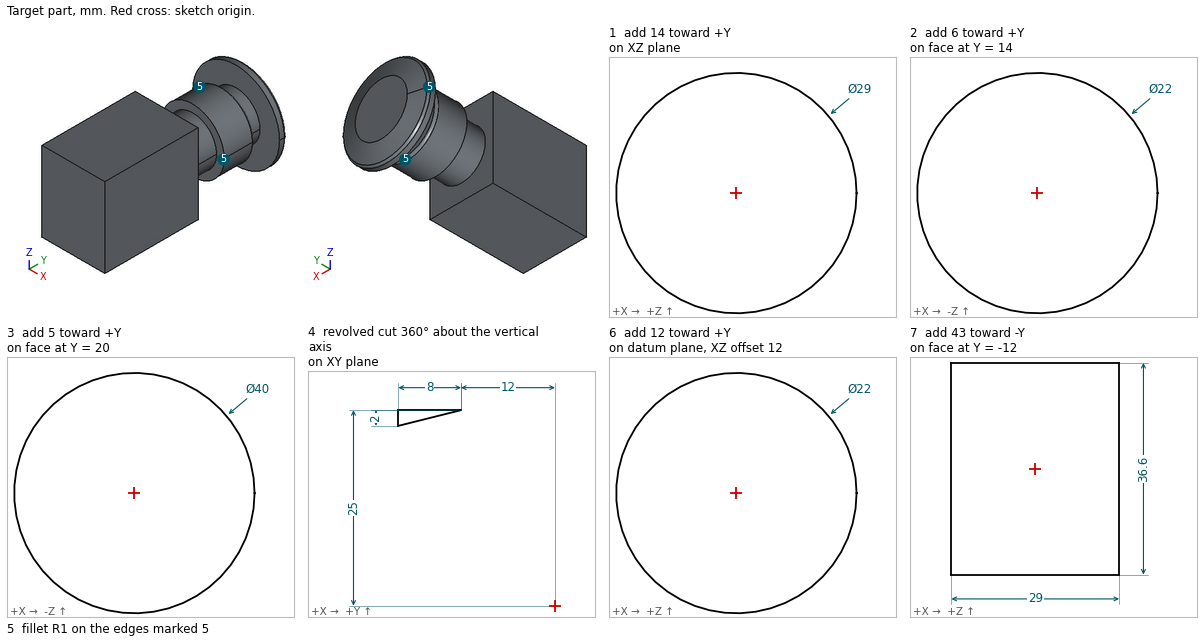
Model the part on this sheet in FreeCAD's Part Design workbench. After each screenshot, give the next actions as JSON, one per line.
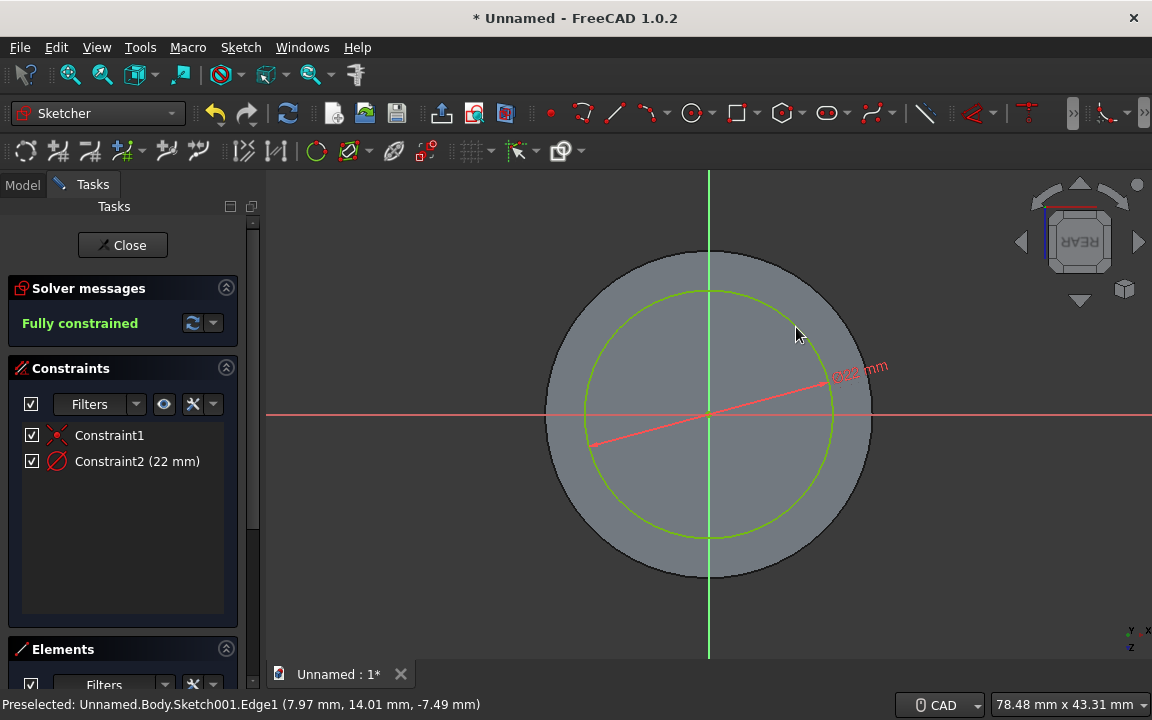
{"action": "left_click", "coordinate": [123, 245]}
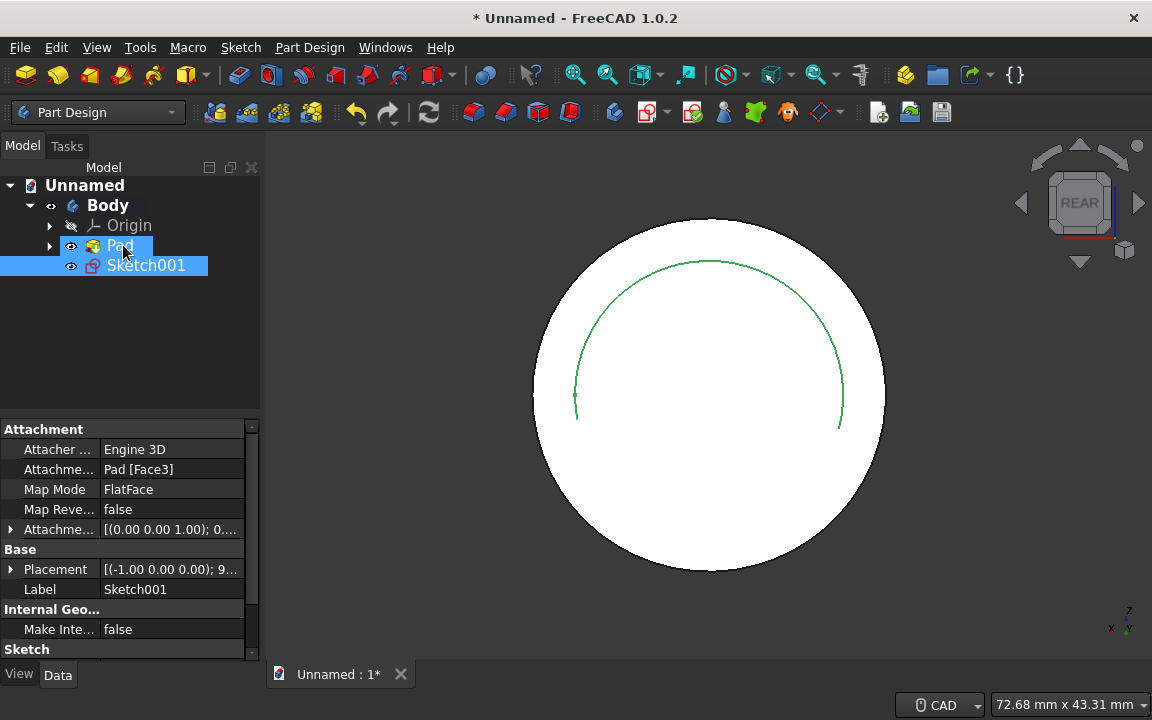
{"action": "left_click", "coordinate": [26, 76]}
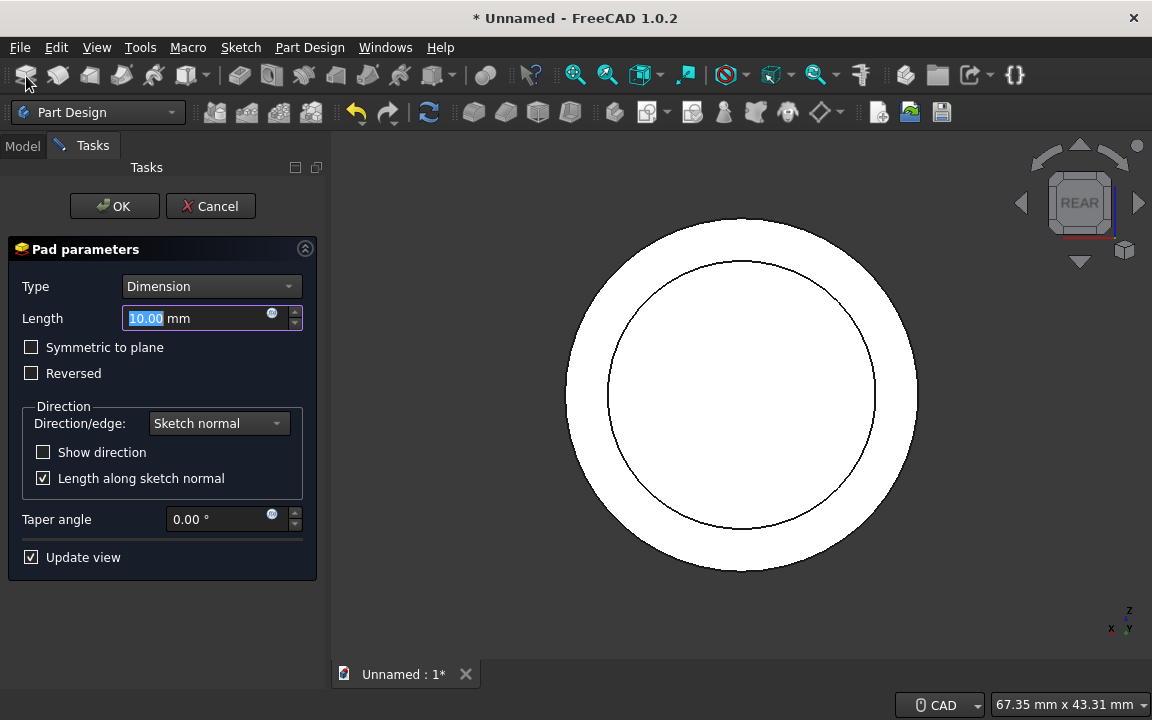
{"action": "type", "text": "6"}
{"action": "key", "text": "Tab"}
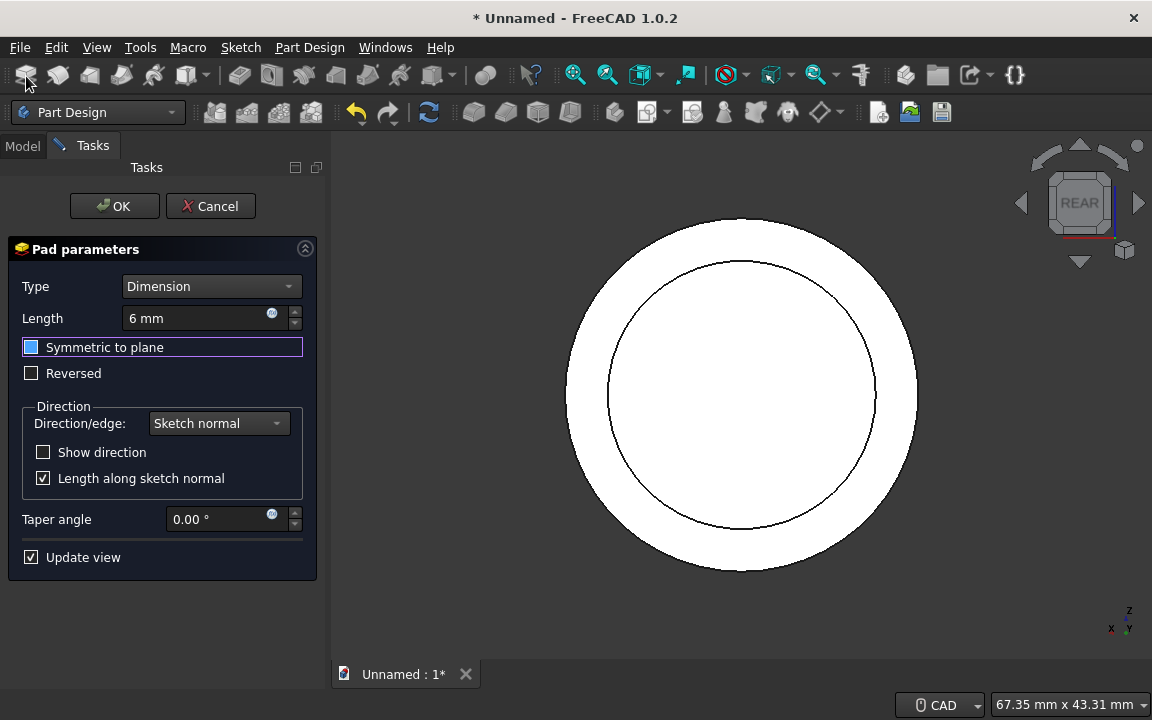
{"action": "left_click", "coordinate": [115, 206]}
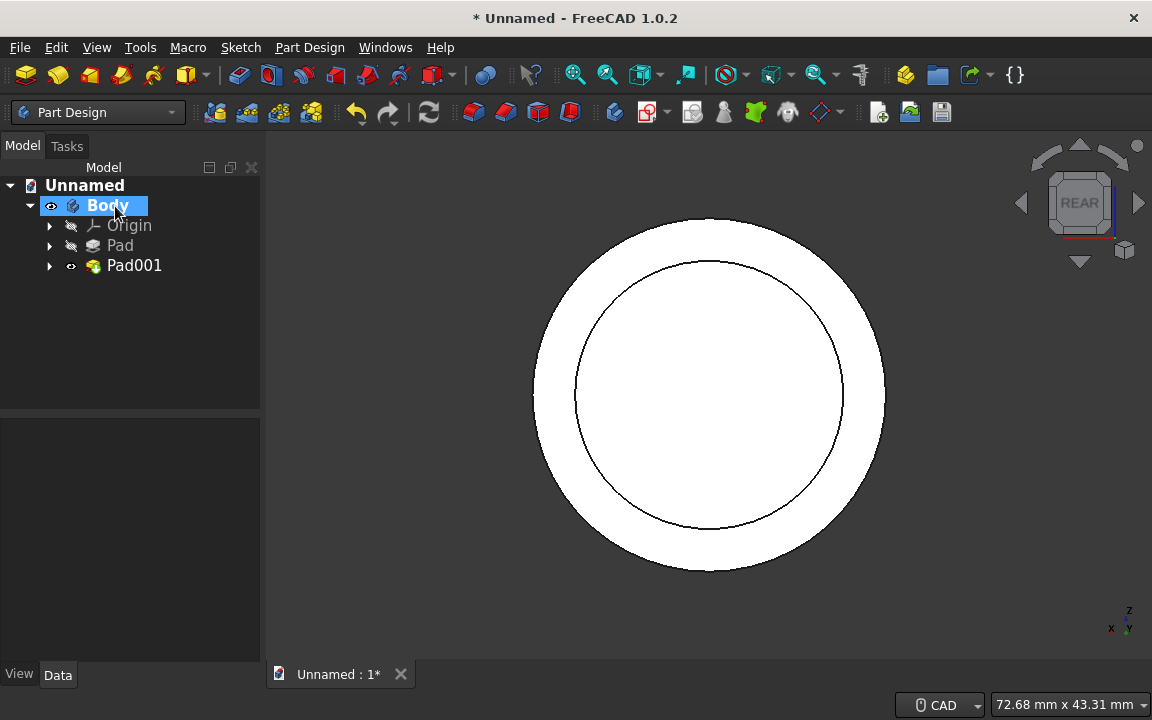
{"action": "left_click", "coordinate": [709, 394]}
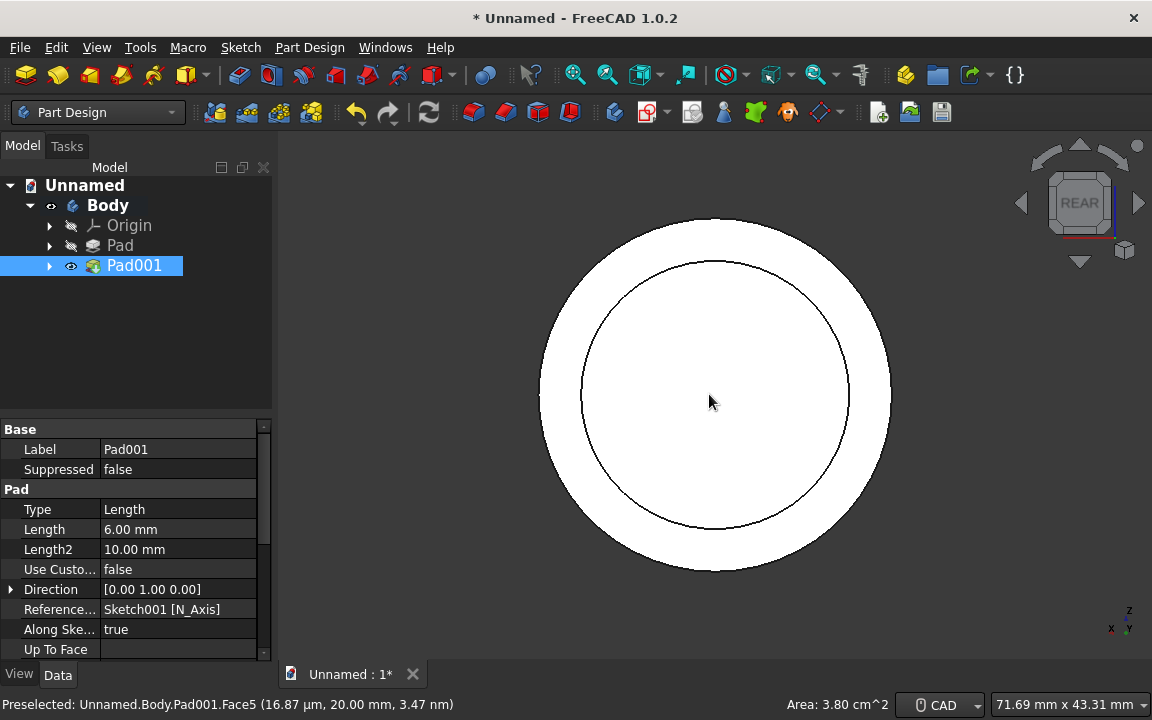
{"action": "left_click", "coordinate": [648, 112]}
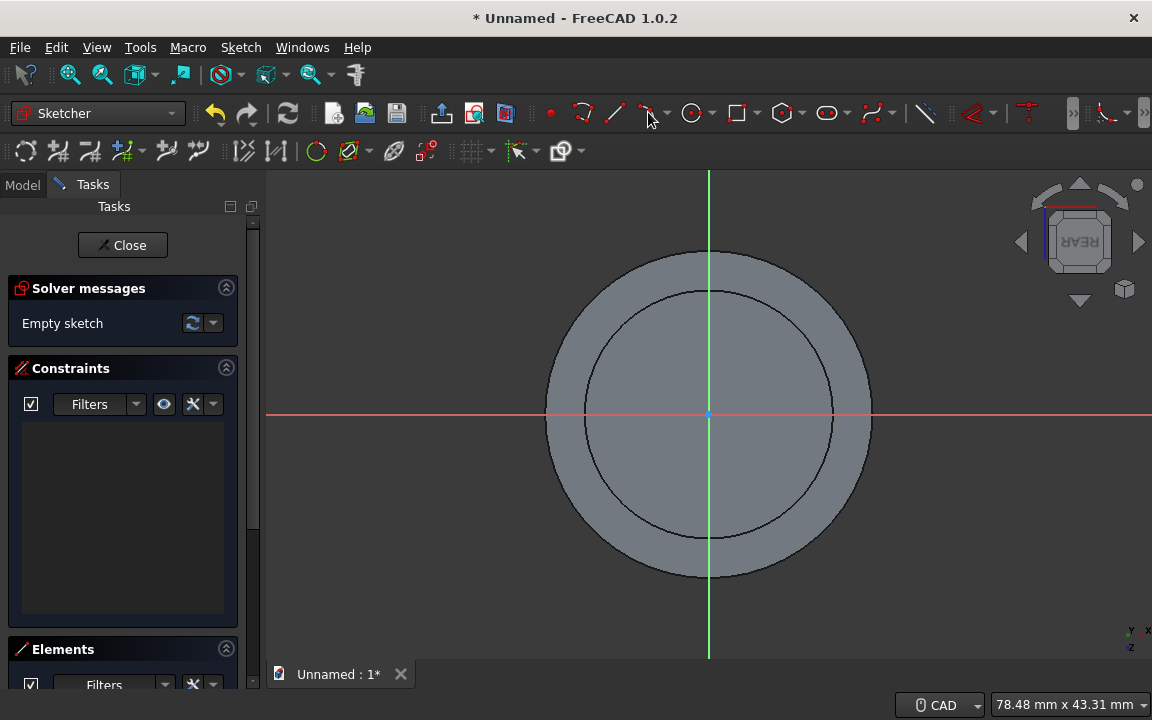
{"action": "scroll", "coordinate": [502, 415], "scroll_direction": "down", "scroll_amount": 2}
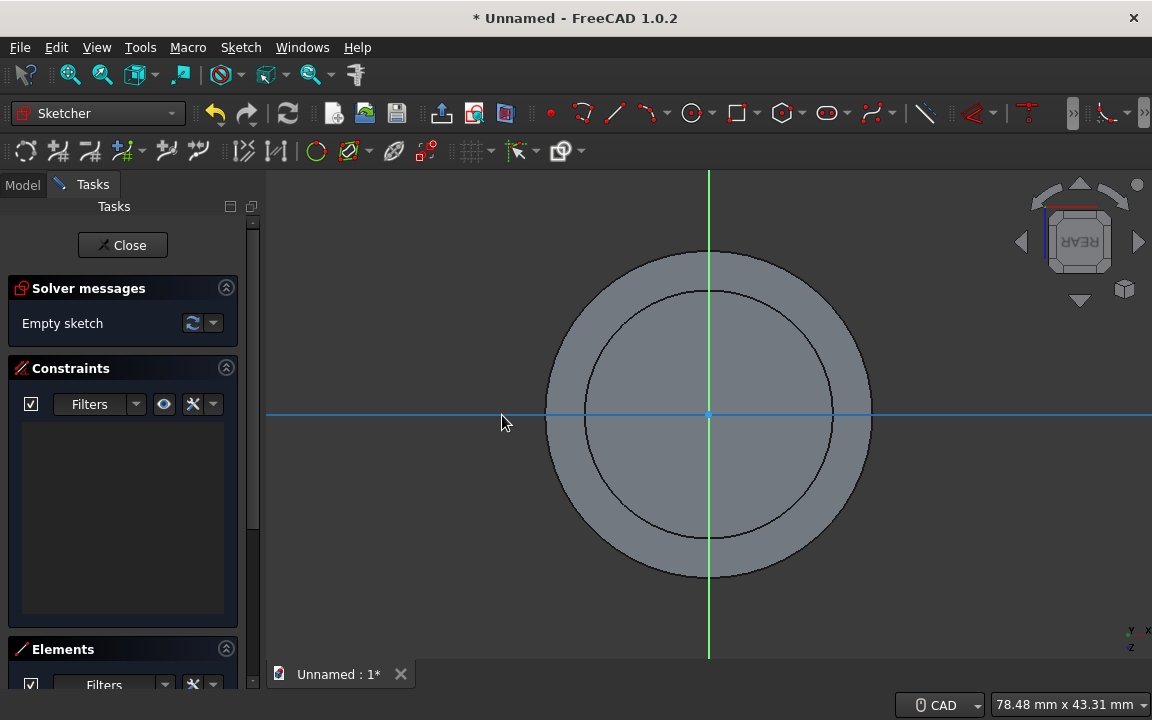
{"action": "key", "text": "g c"}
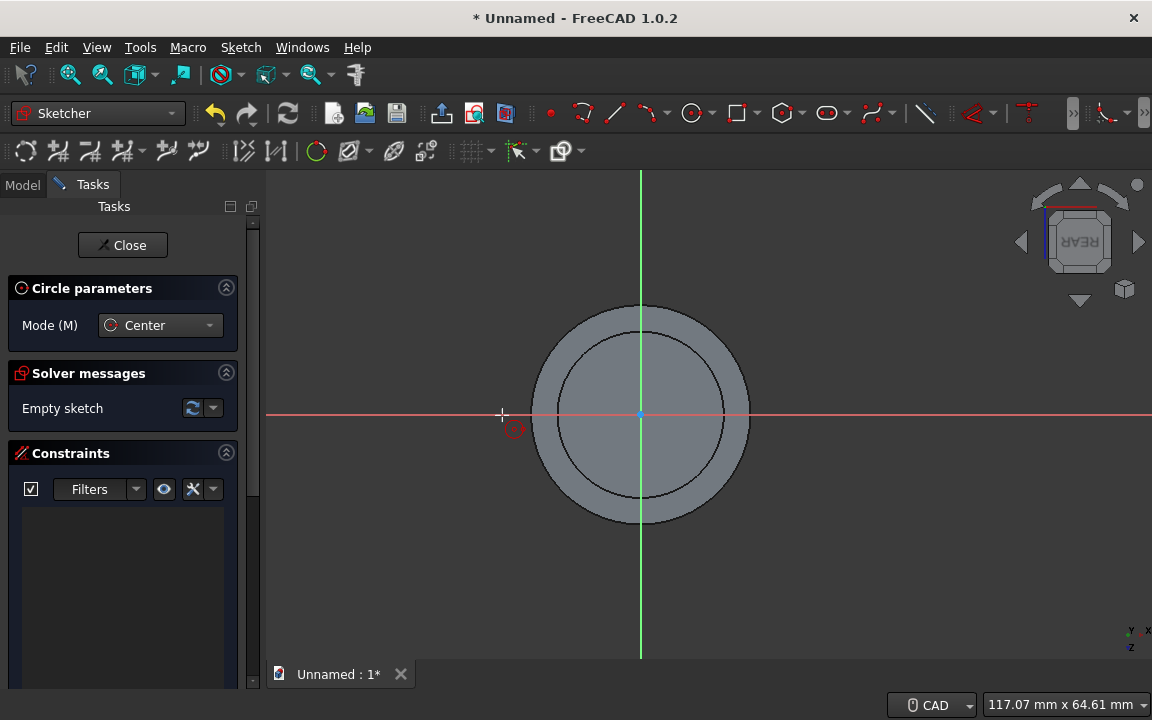
{"action": "left_click", "coordinate": [641, 415]}
{"action": "left_click", "coordinate": [748, 308]}
{"action": "key", "text": "Escape"}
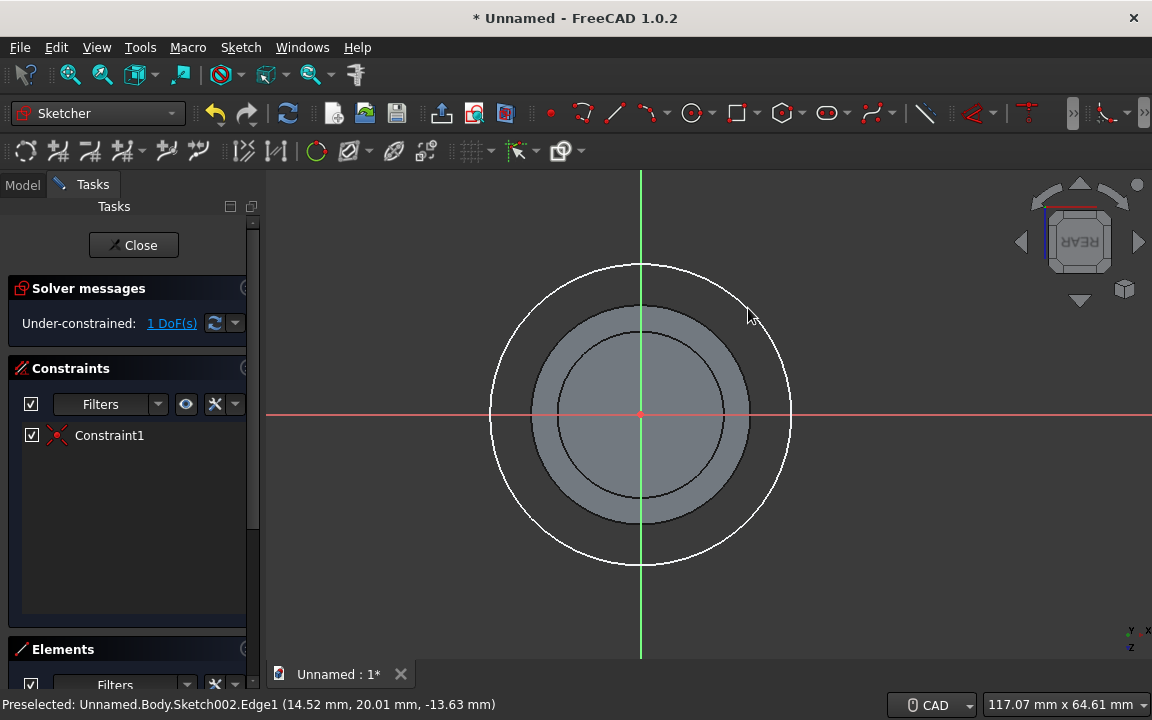
{"action": "left_click", "coordinate": [747, 308]}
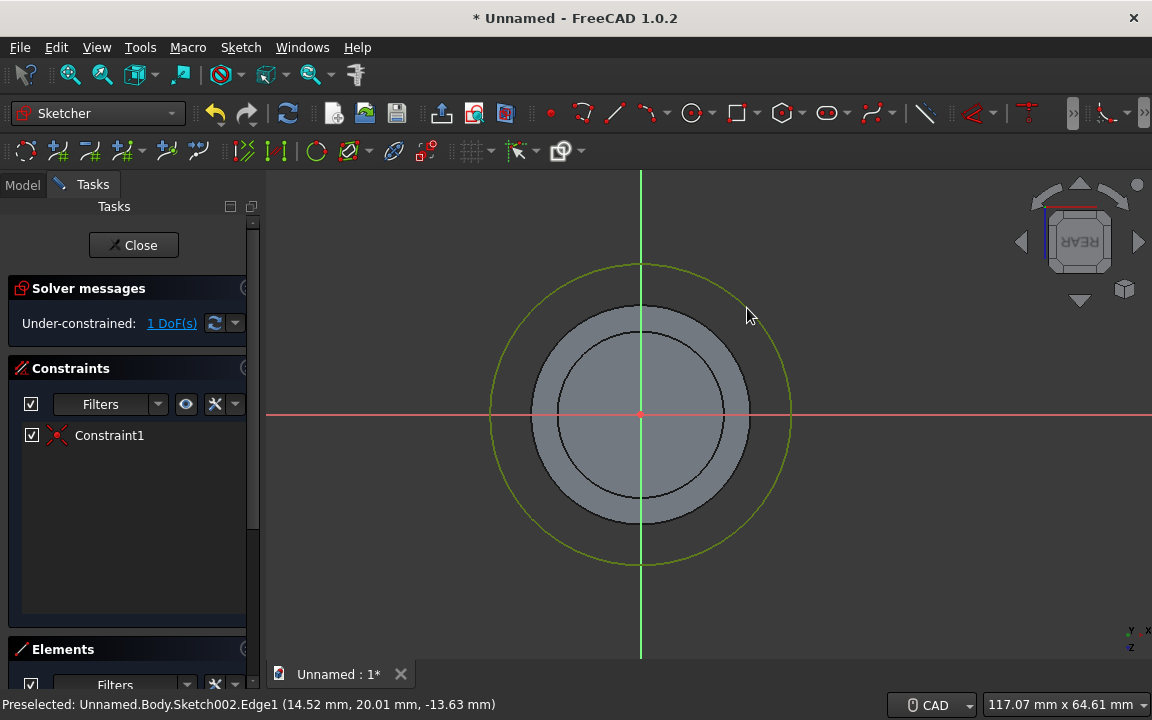
{"action": "key", "text": "k o"}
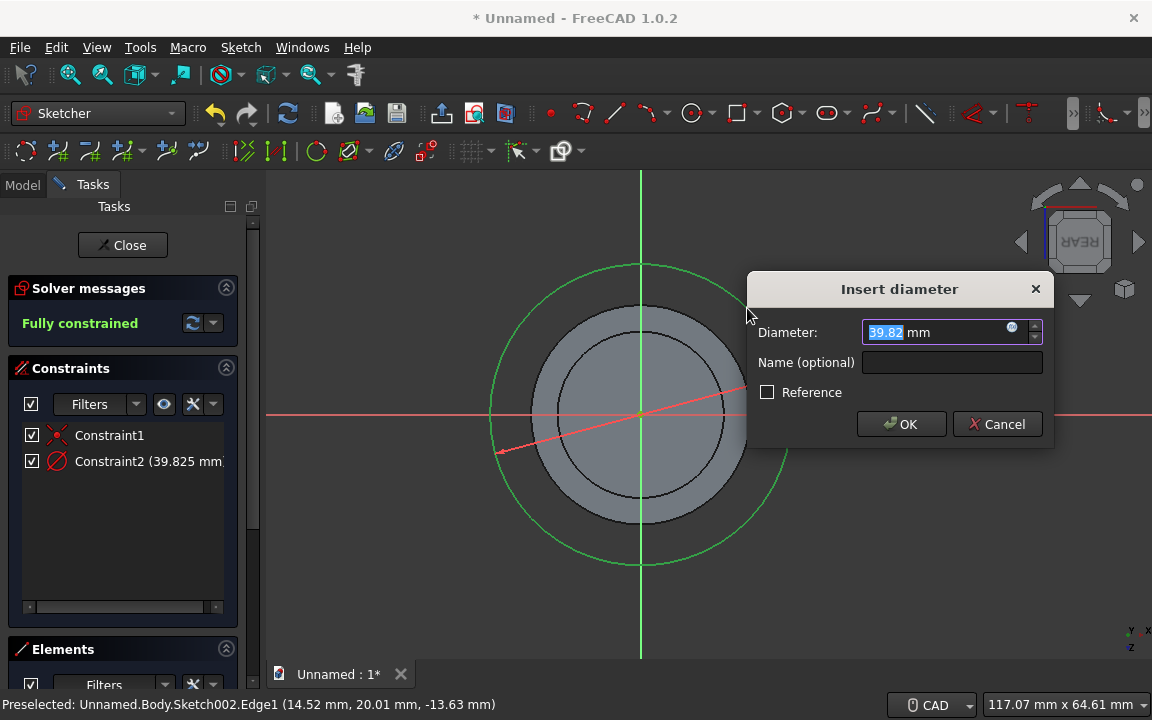
{"action": "type", "text": "40"}
{"action": "key", "text": "Return"}